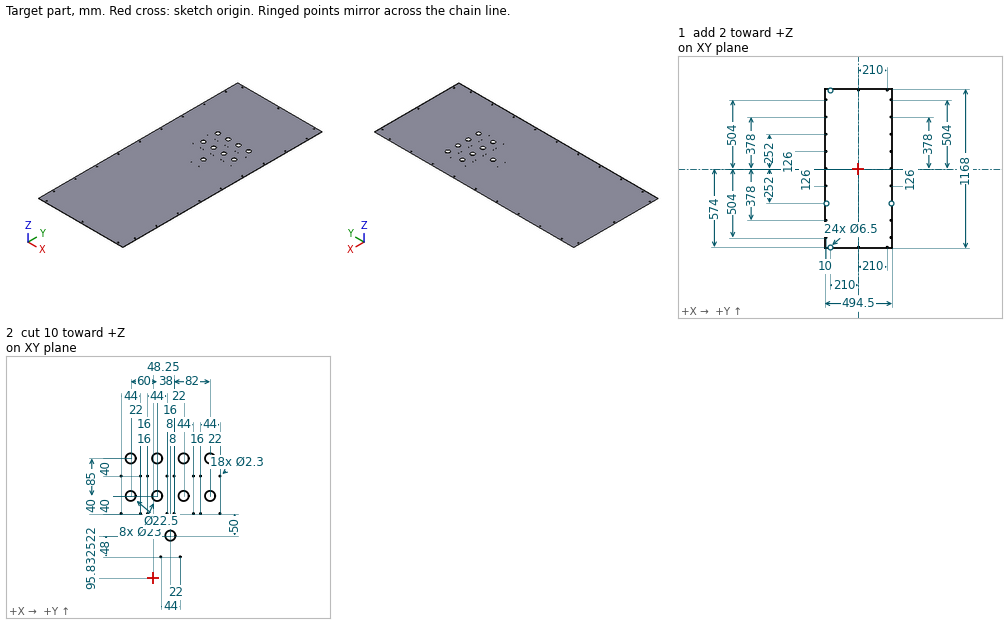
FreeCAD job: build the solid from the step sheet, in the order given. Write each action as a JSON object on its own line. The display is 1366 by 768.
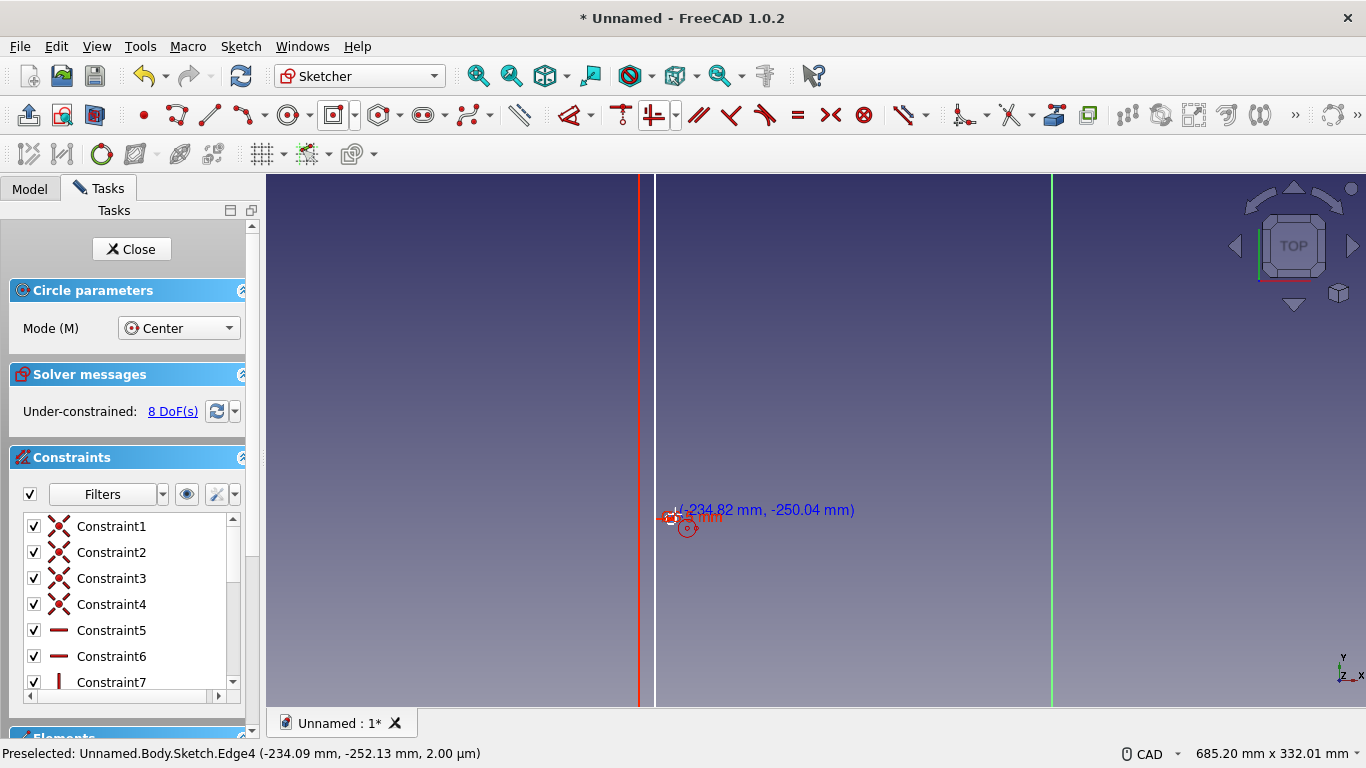
{"action": "scroll", "coordinate": [671, 316], "scroll_direction": "up", "scroll_amount": 8}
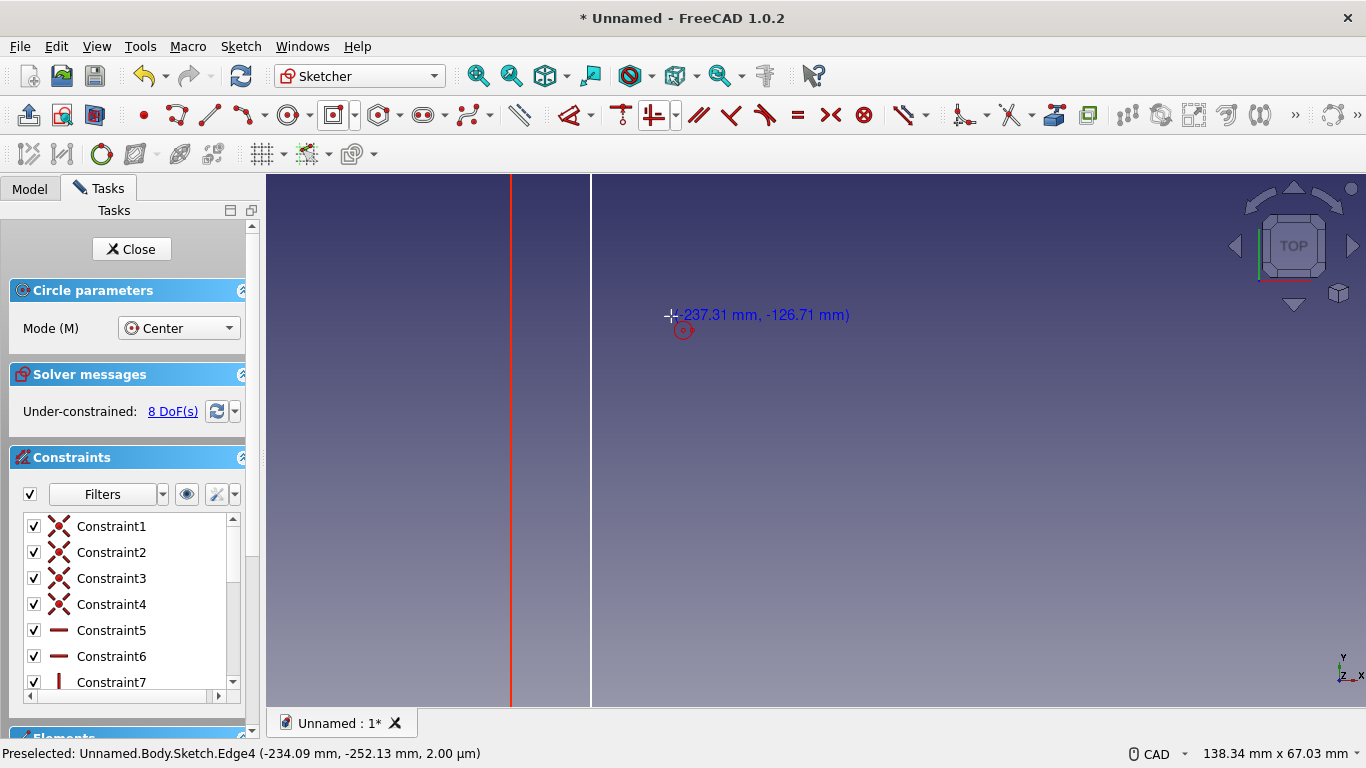
{"action": "scroll", "coordinate": [671, 488], "scroll_direction": "down", "scroll_amount": 16}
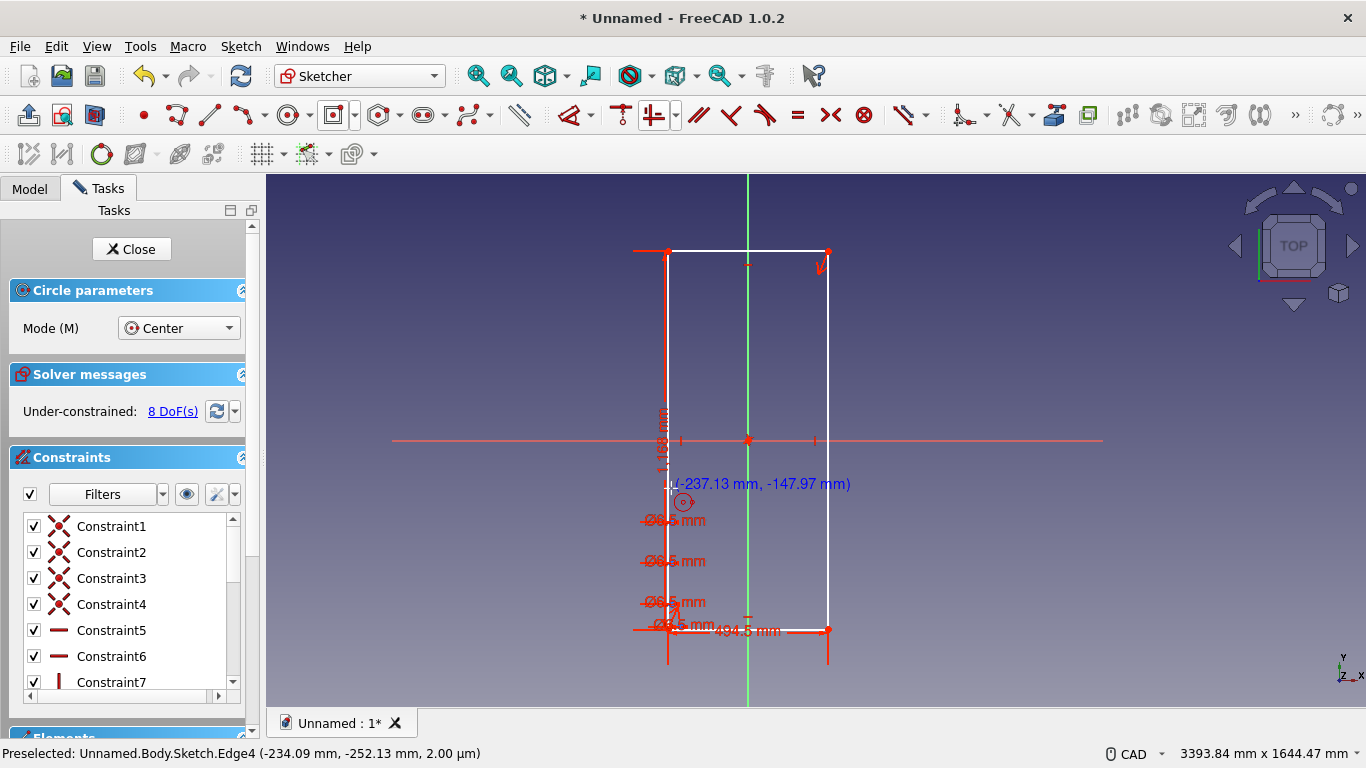
{"action": "scroll", "coordinate": [671, 481], "scroll_direction": "up", "scroll_amount": 8}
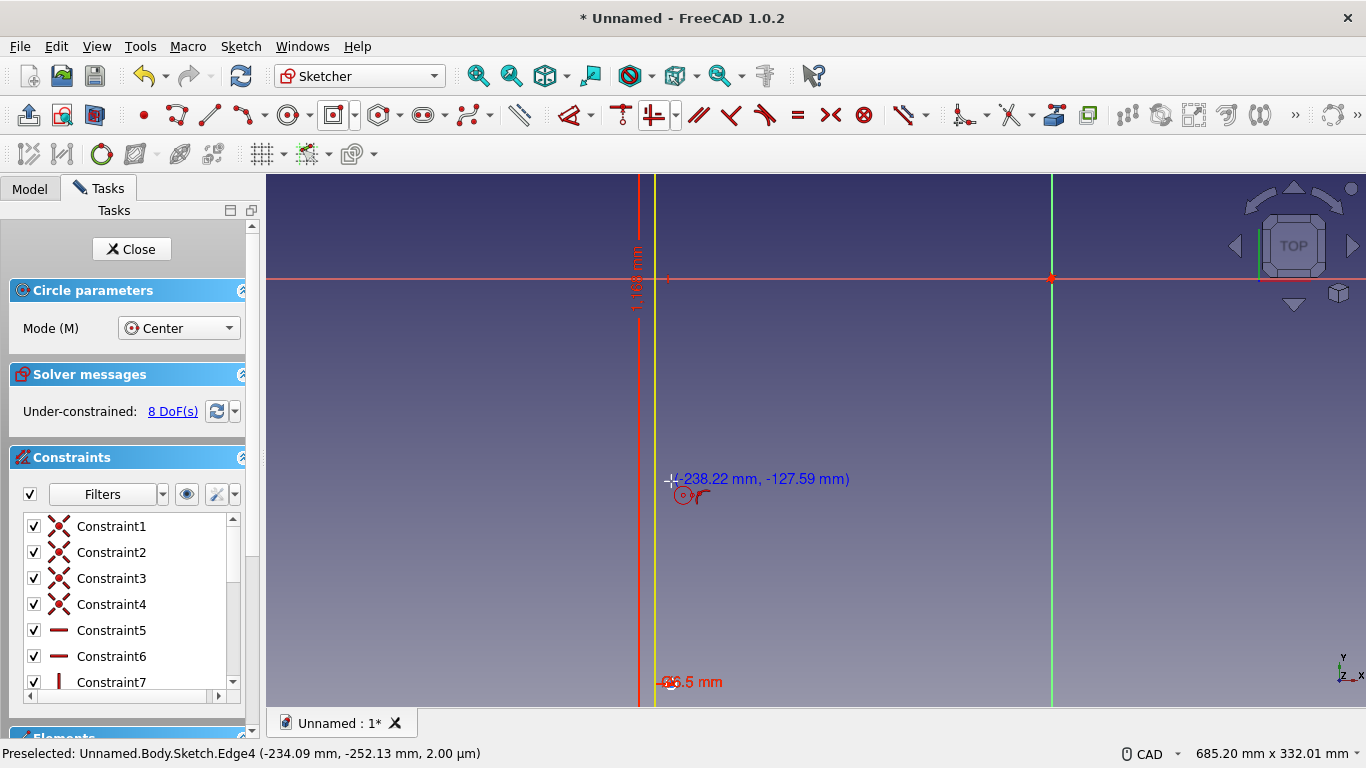
{"action": "left_click", "coordinate": [671, 481]}
{"action": "mouse_move", "coordinate": [675, 477]}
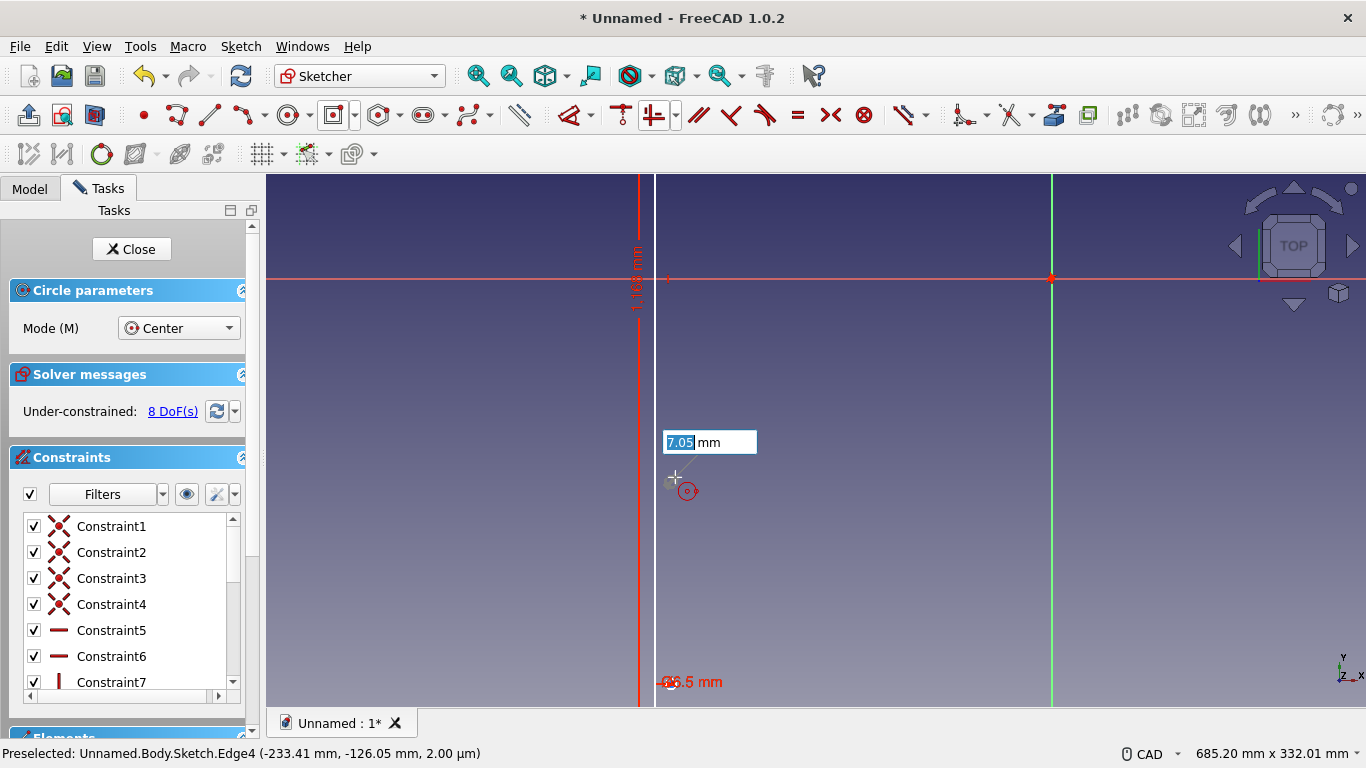
{"action": "type", "text": "6.5"}
{"action": "key", "text": "Return"}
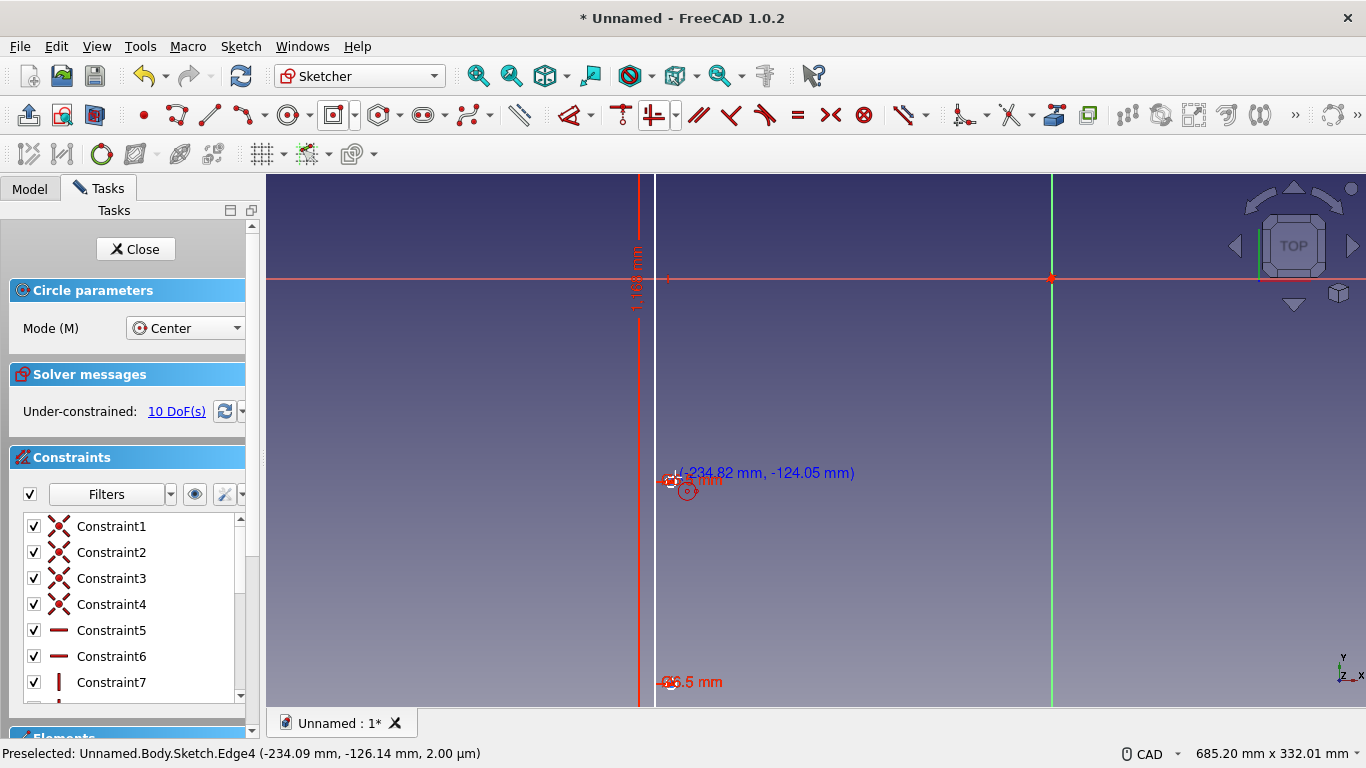
{"action": "scroll", "coordinate": [687, 473], "scroll_direction": "down", "scroll_amount": 9}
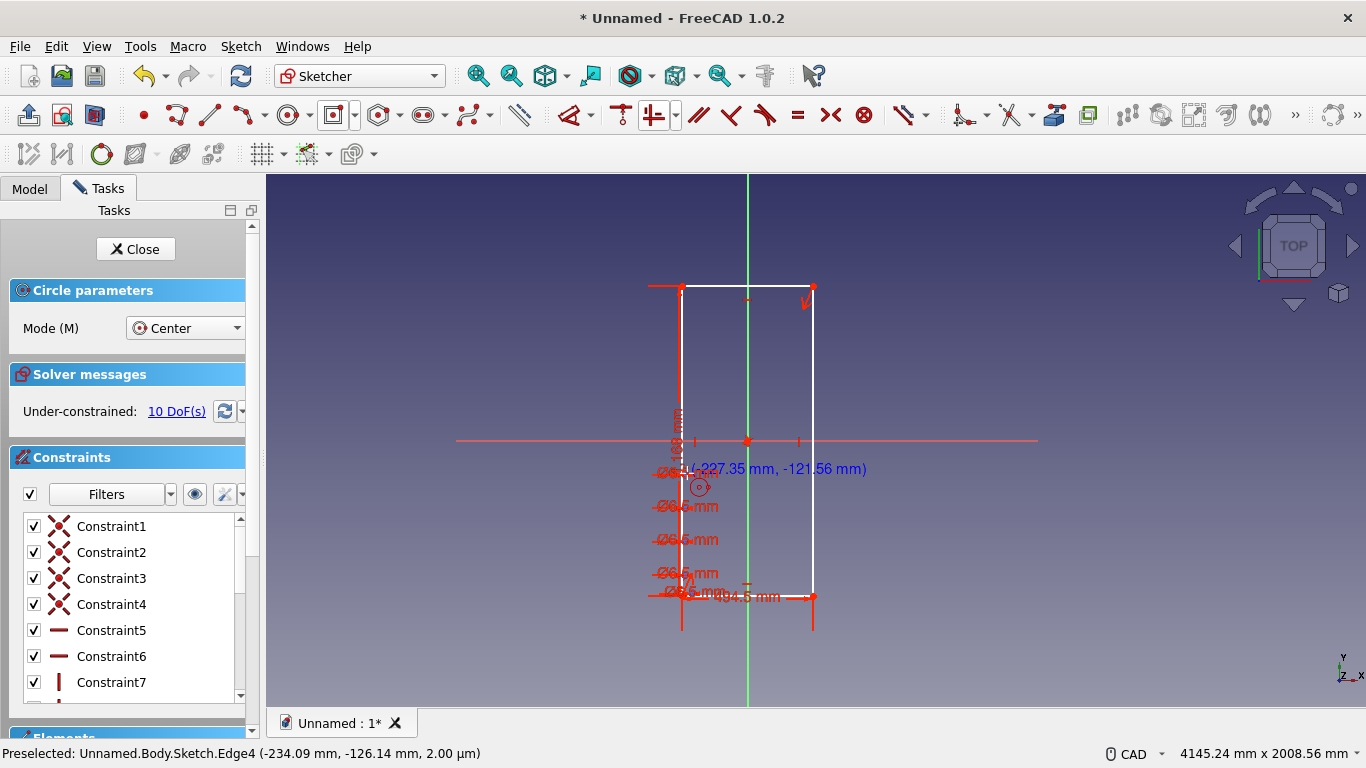
{"action": "scroll", "coordinate": [748, 594], "scroll_direction": "up", "scroll_amount": 17}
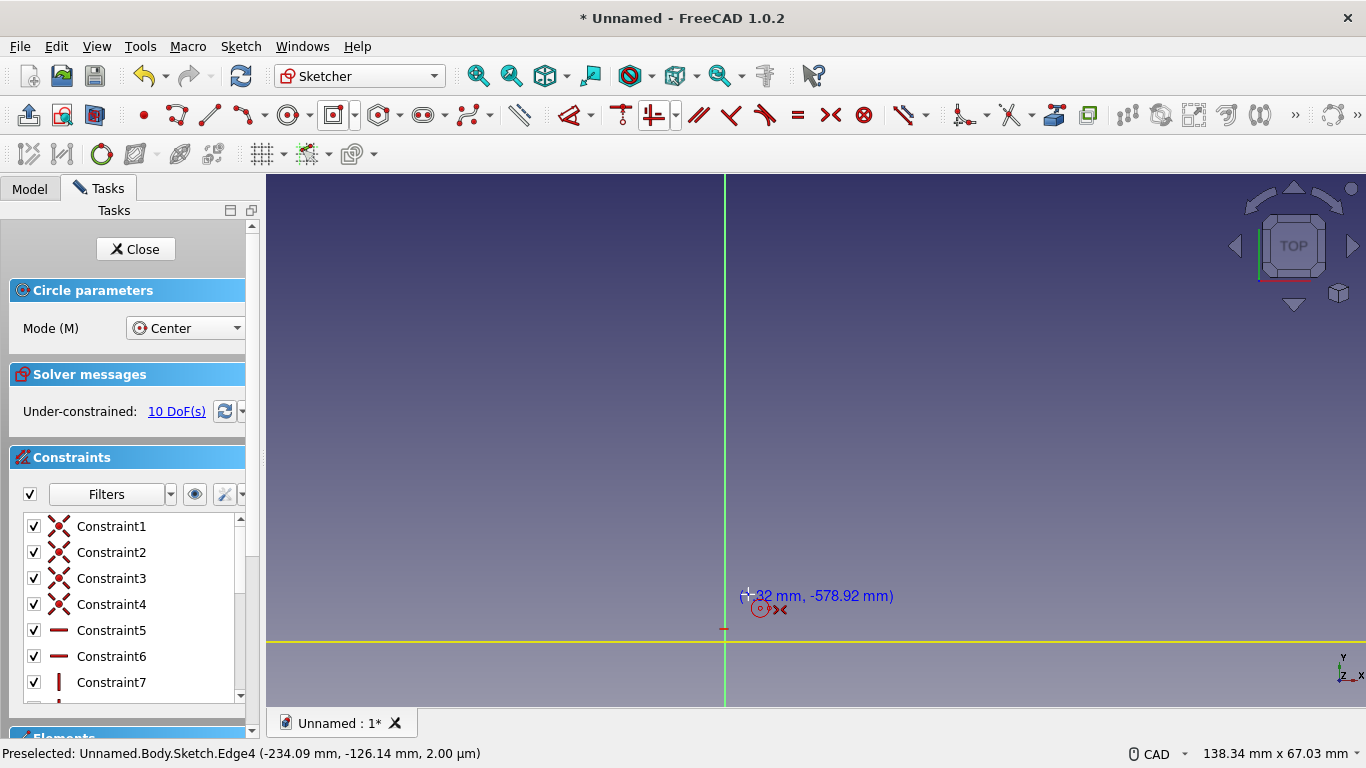
{"action": "scroll", "coordinate": [748, 629], "scroll_direction": "down", "scroll_amount": 16}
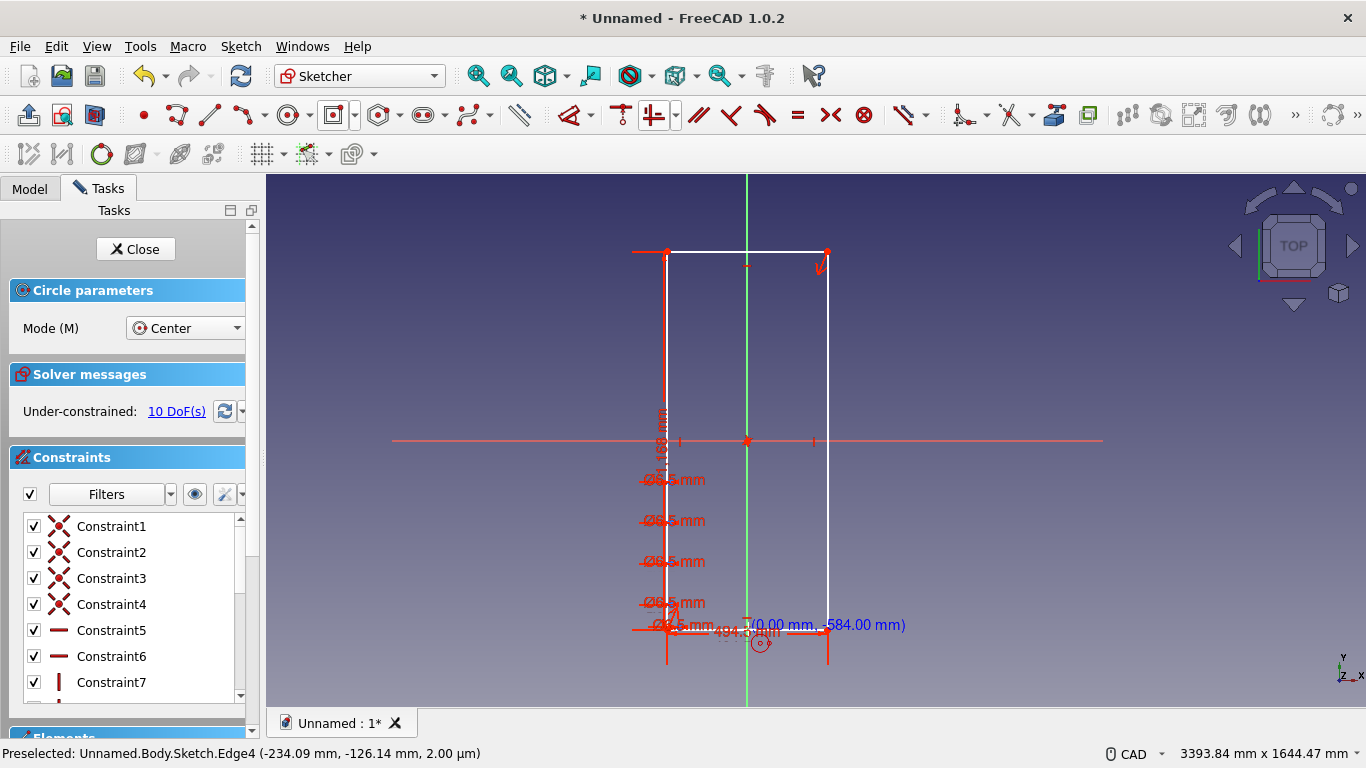
{"action": "scroll", "coordinate": [747, 627], "scroll_direction": "up", "scroll_amount": 8}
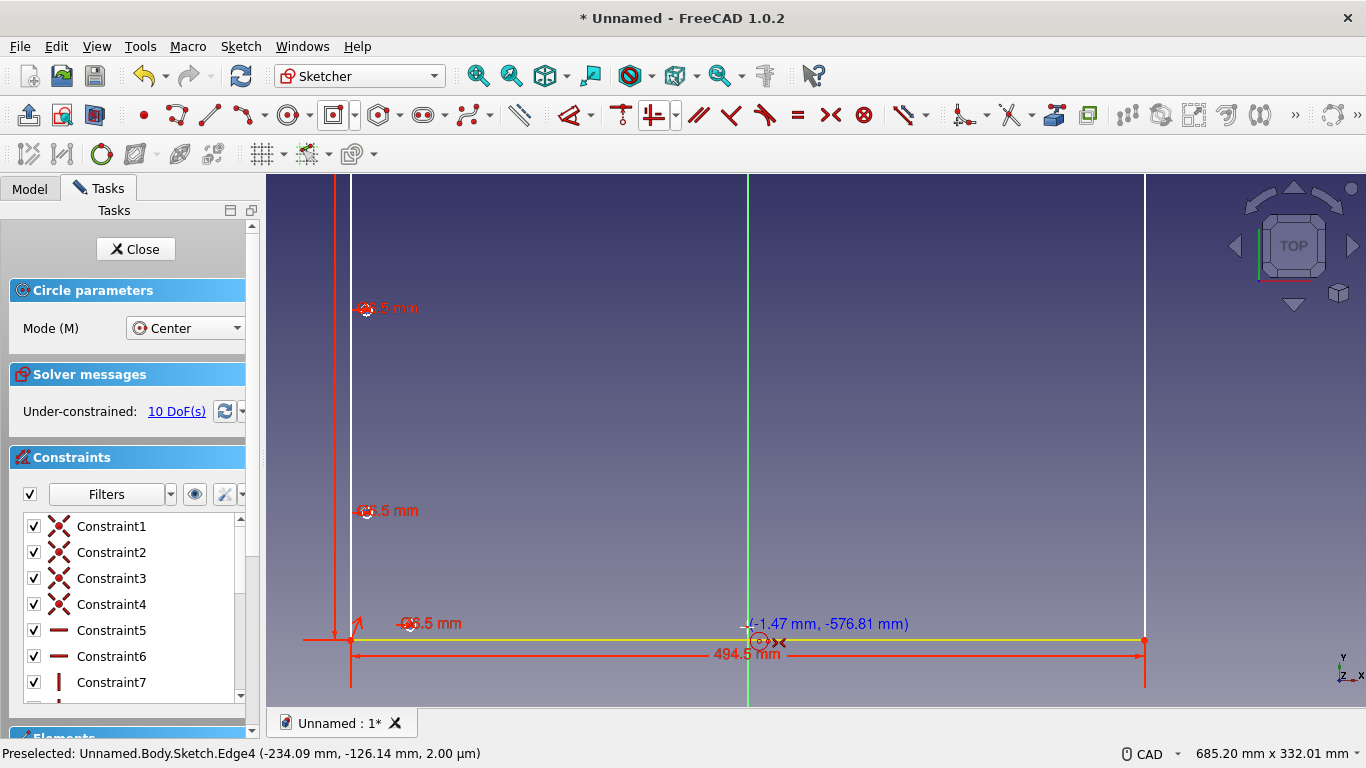
{"action": "left_click", "coordinate": [748, 624]}